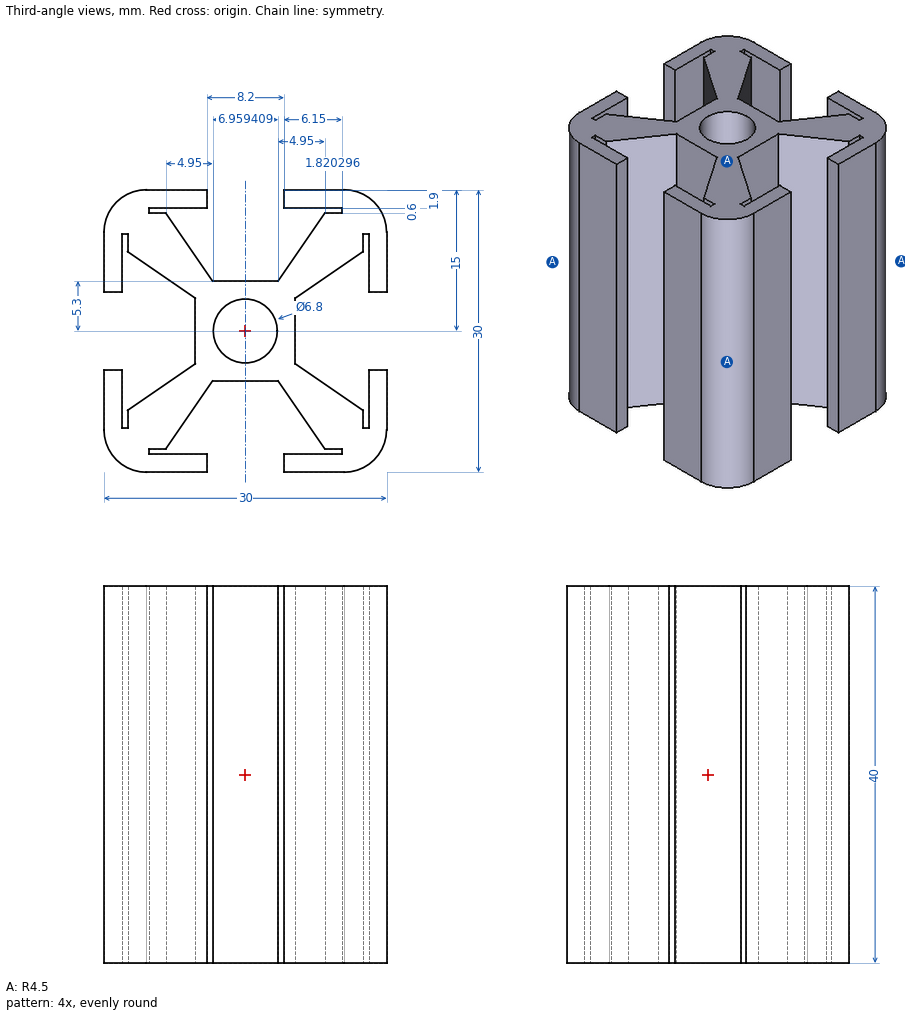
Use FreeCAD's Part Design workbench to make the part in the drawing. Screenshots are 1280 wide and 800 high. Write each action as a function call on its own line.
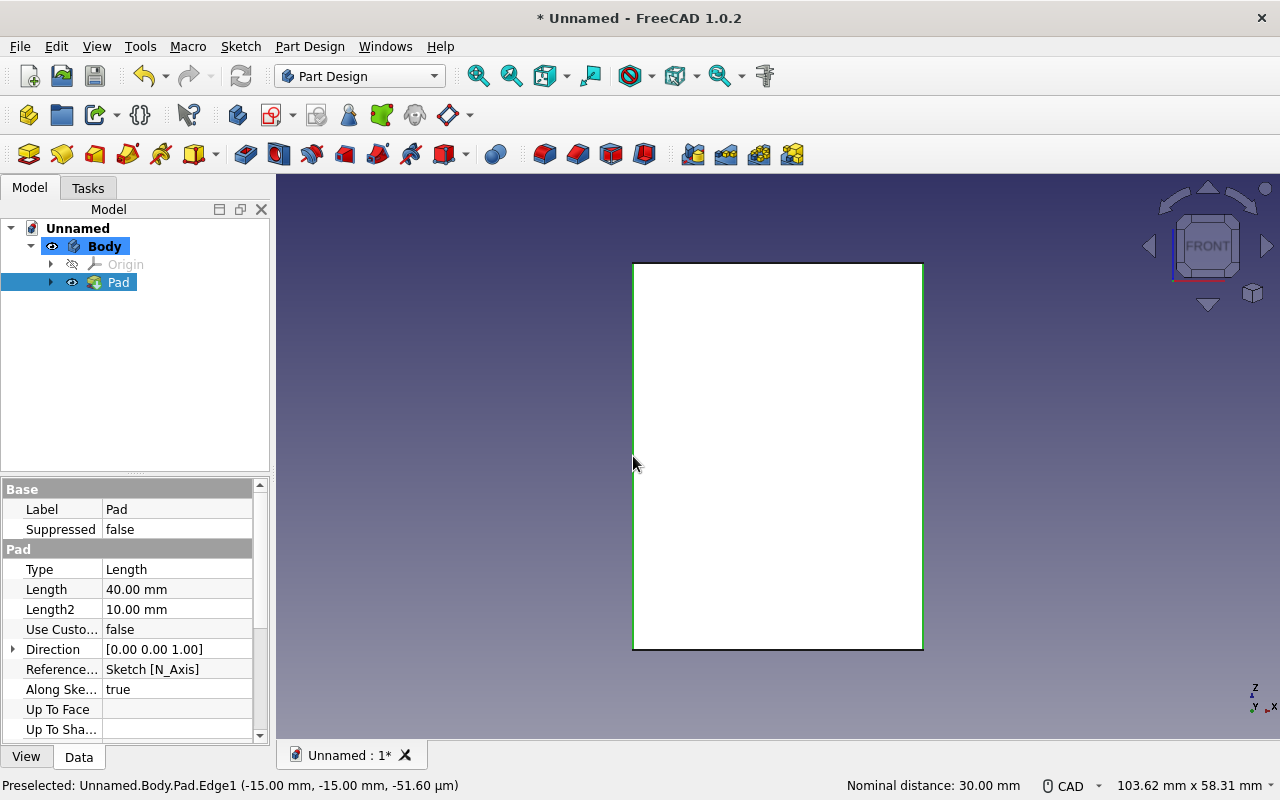
click(923, 455, ctrl)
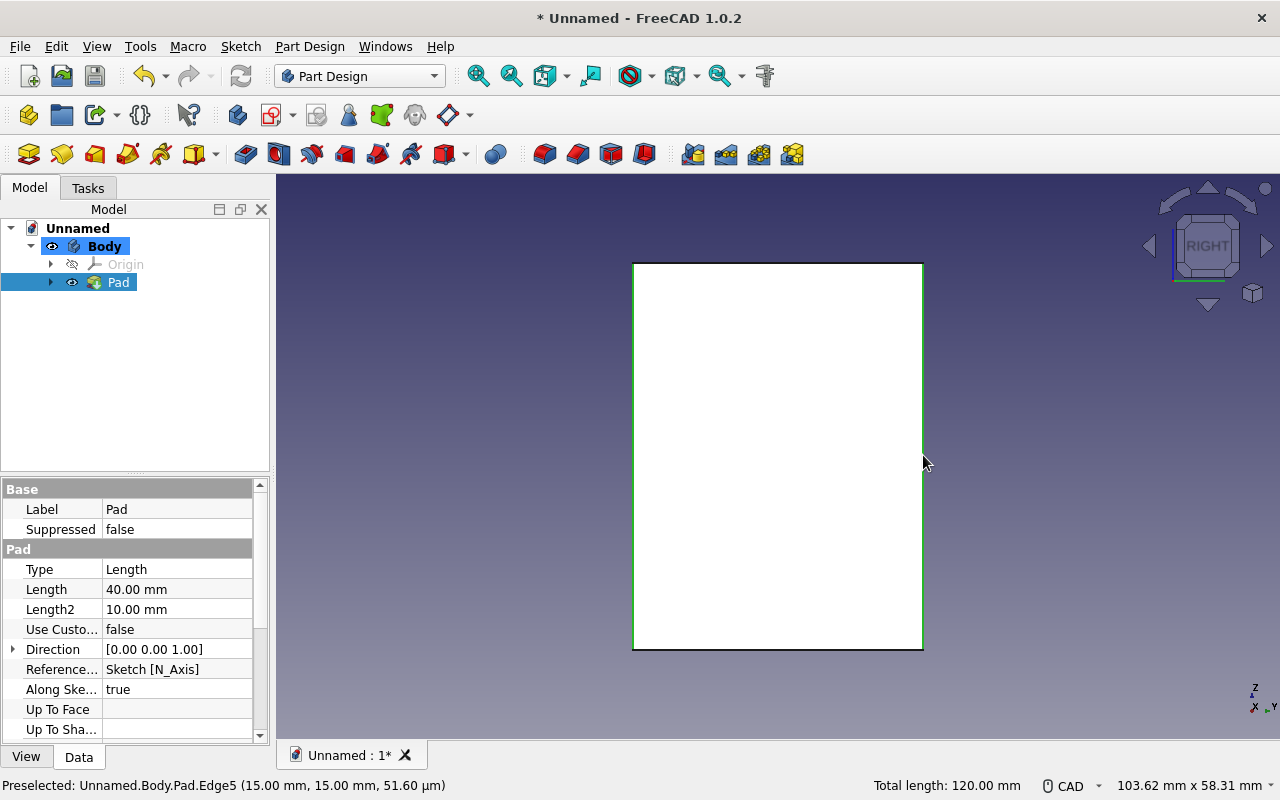
key(5)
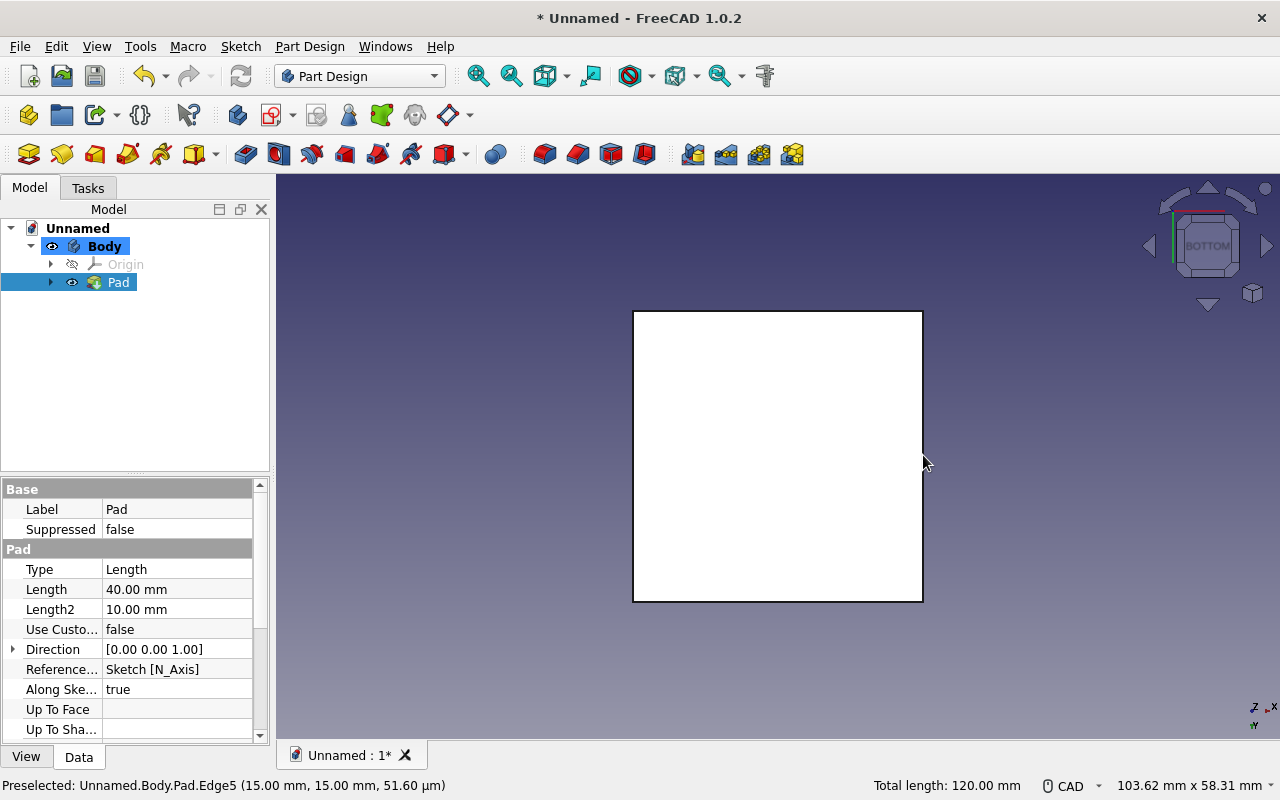
key(4)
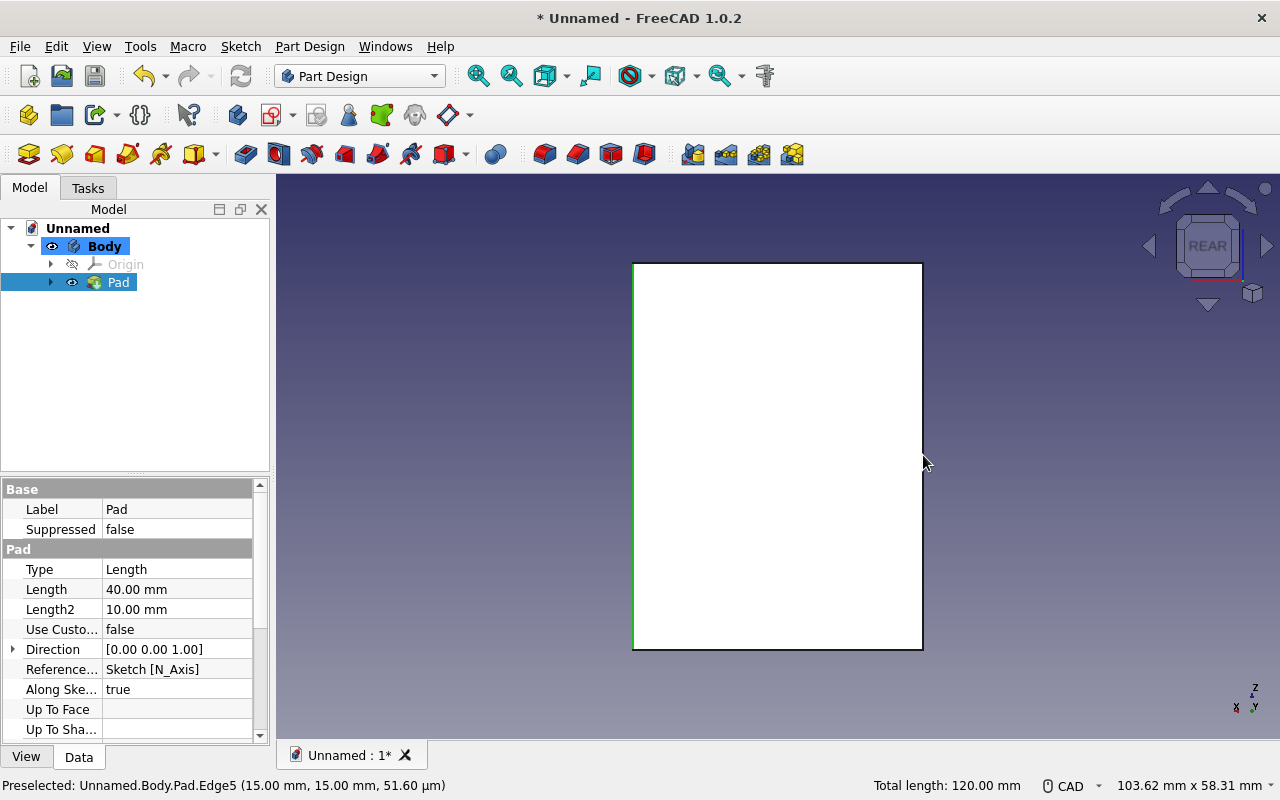
click(923, 456, ctrl)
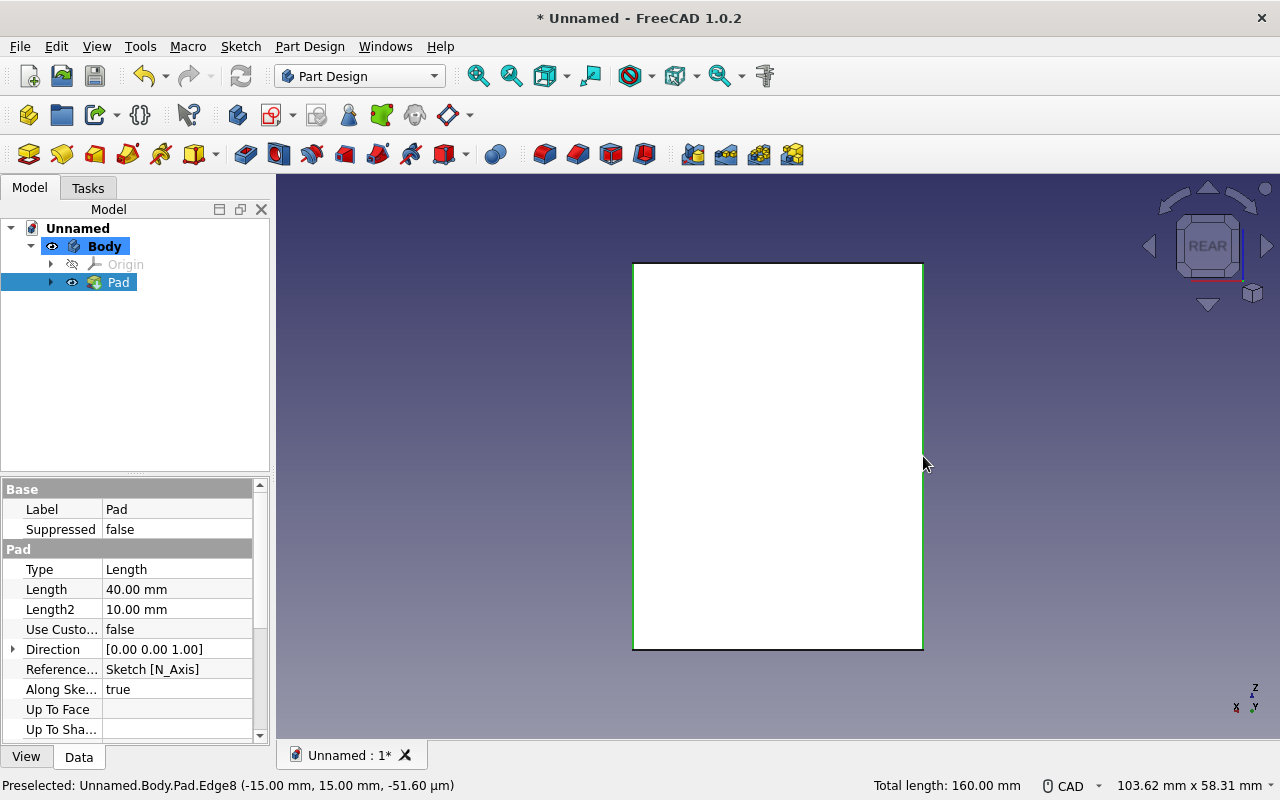
click(545, 154)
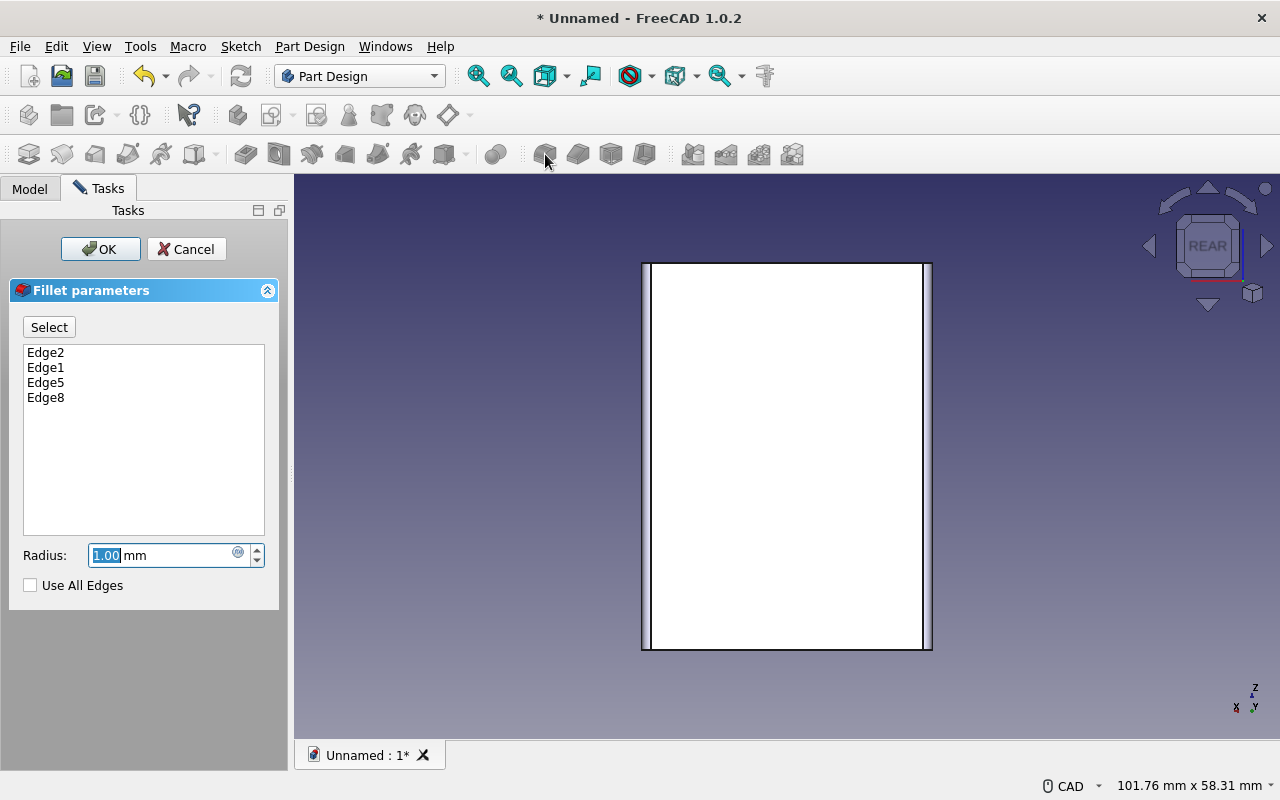
text(4.5)
key(Tab)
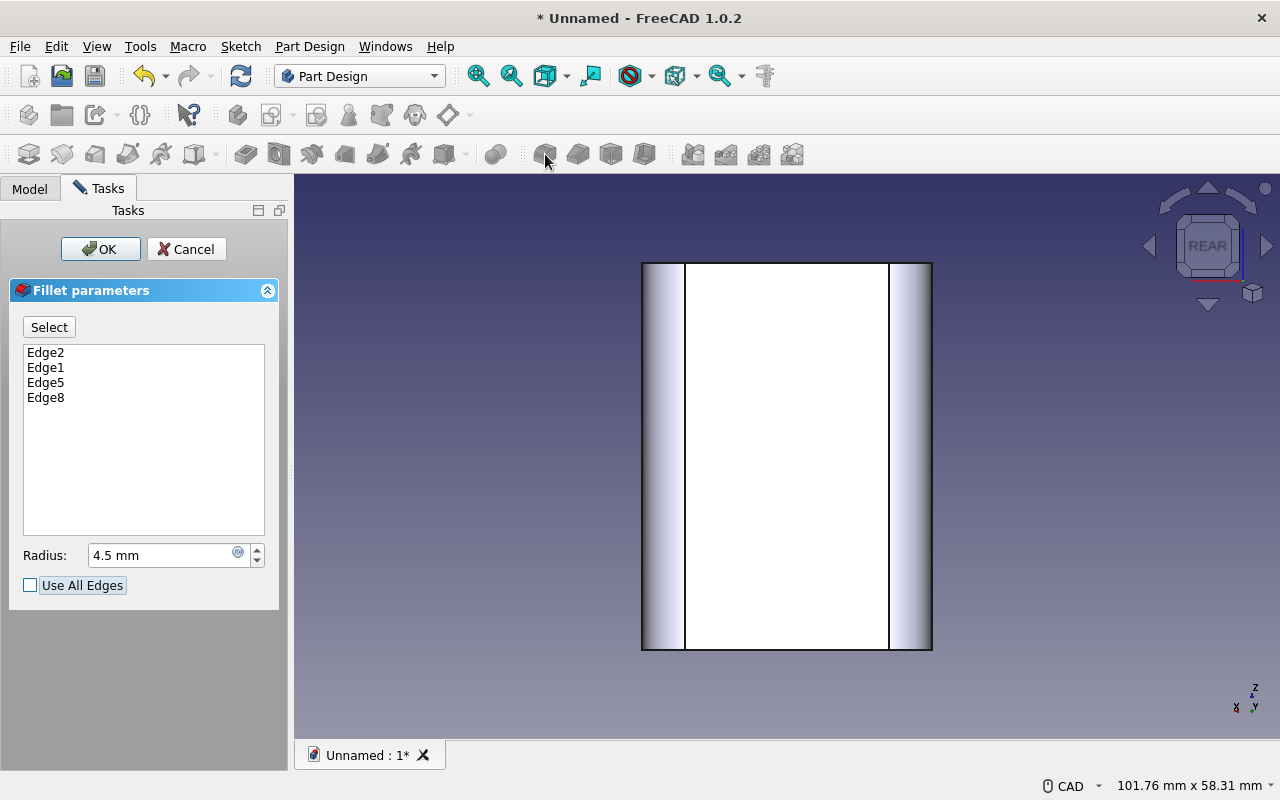
click(101, 249)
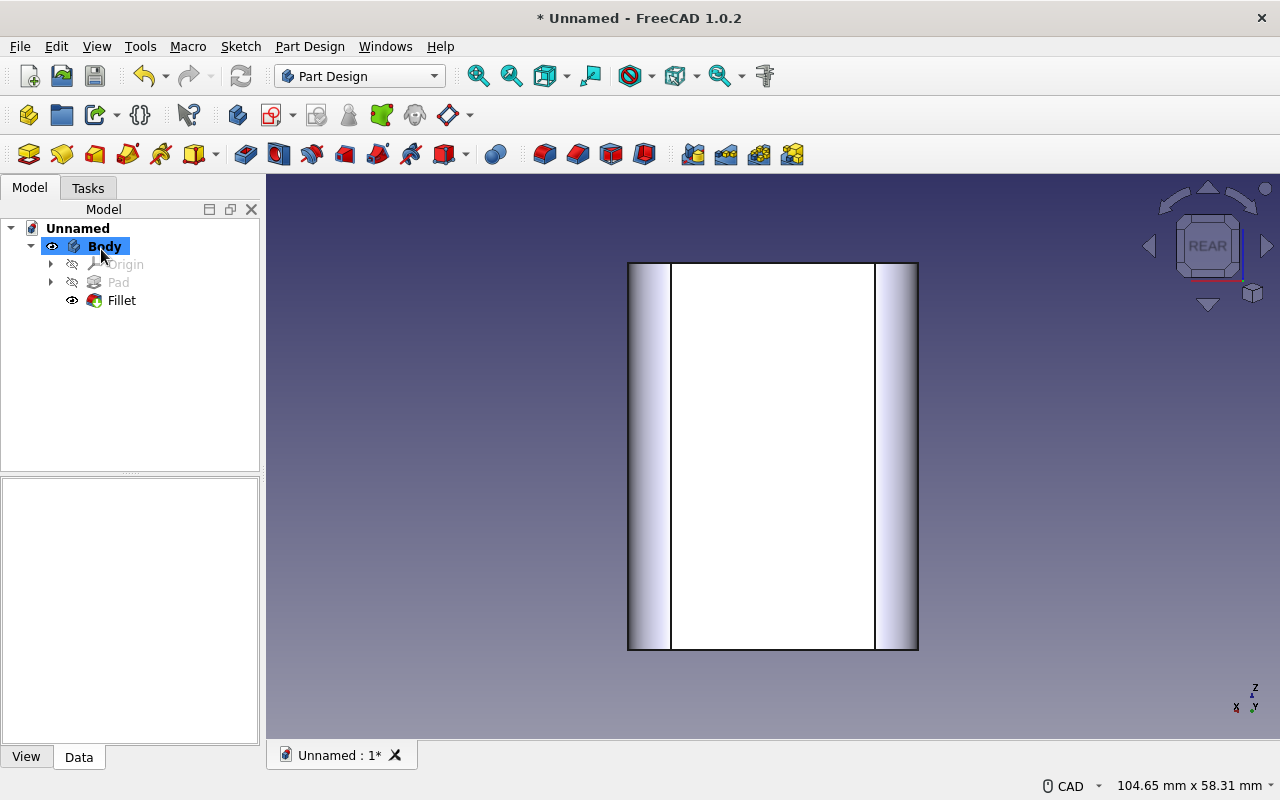
key(0)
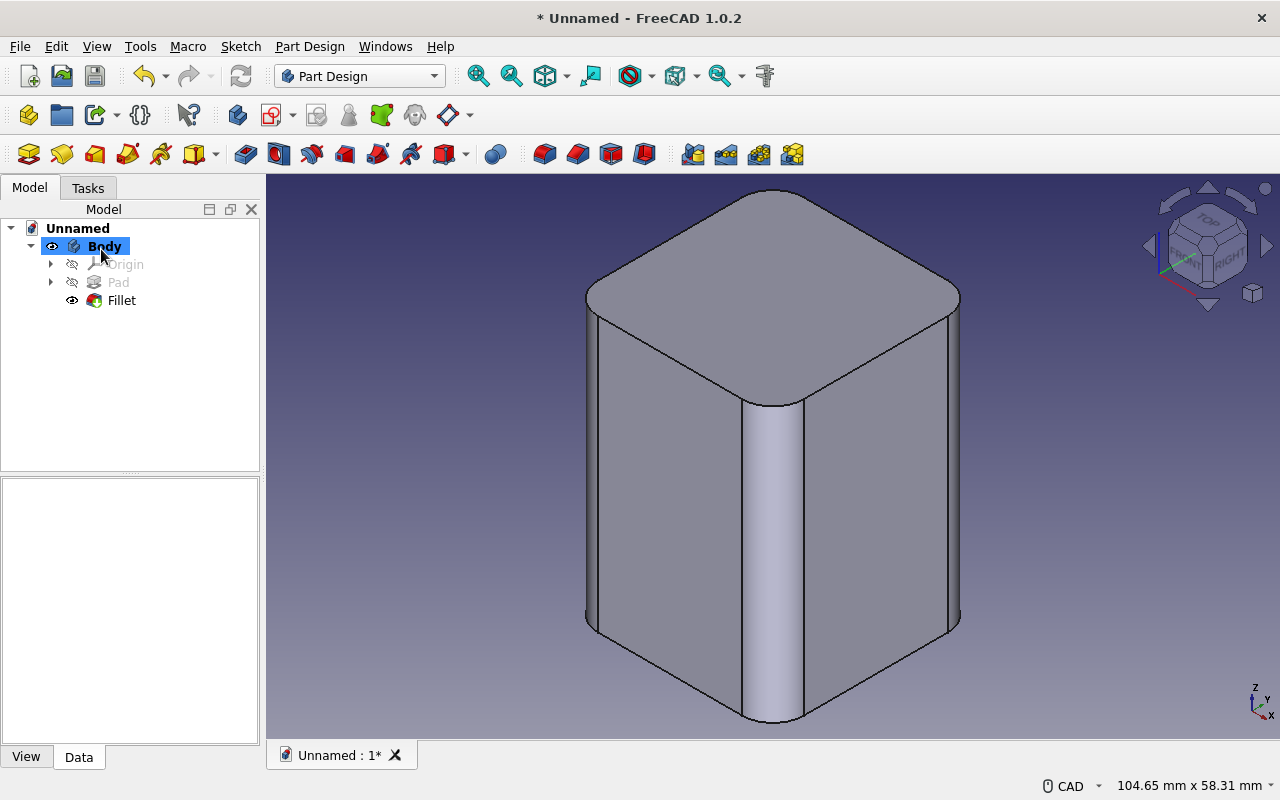
click(773, 297)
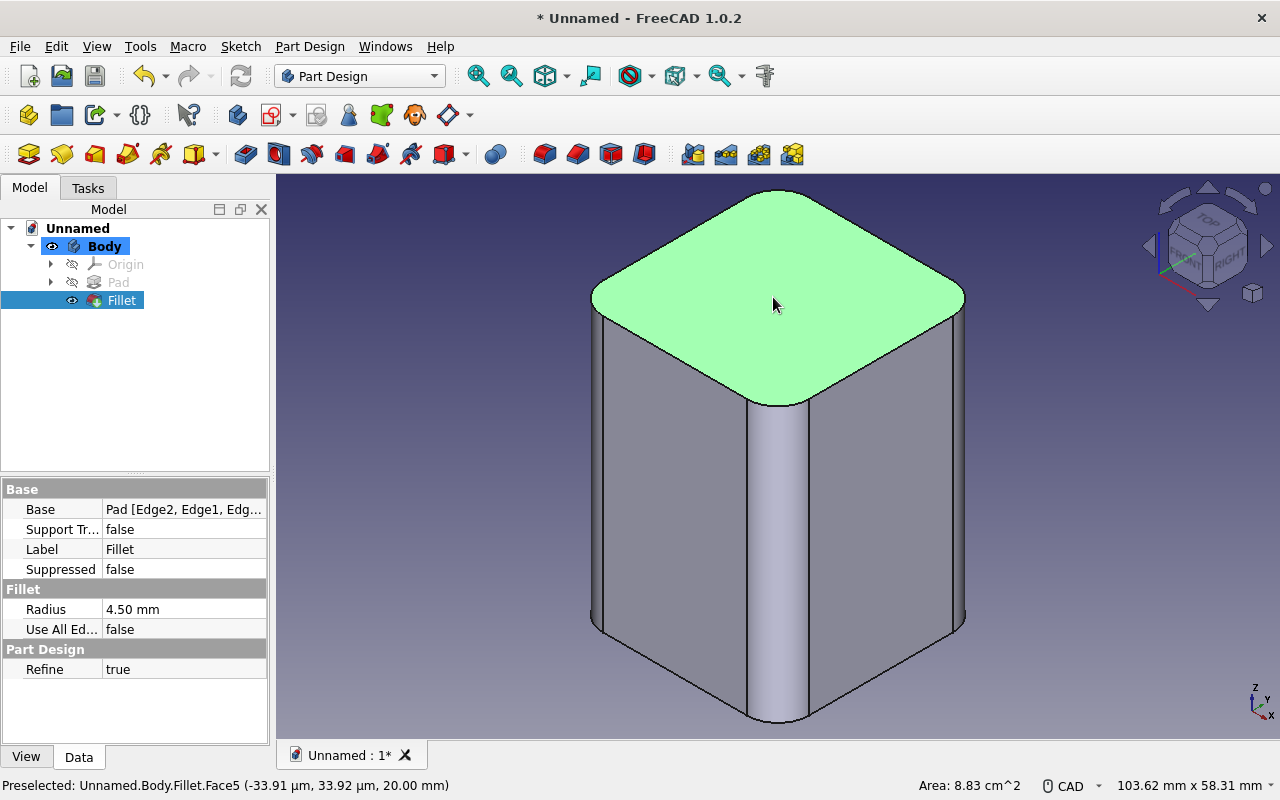
click(270, 116)